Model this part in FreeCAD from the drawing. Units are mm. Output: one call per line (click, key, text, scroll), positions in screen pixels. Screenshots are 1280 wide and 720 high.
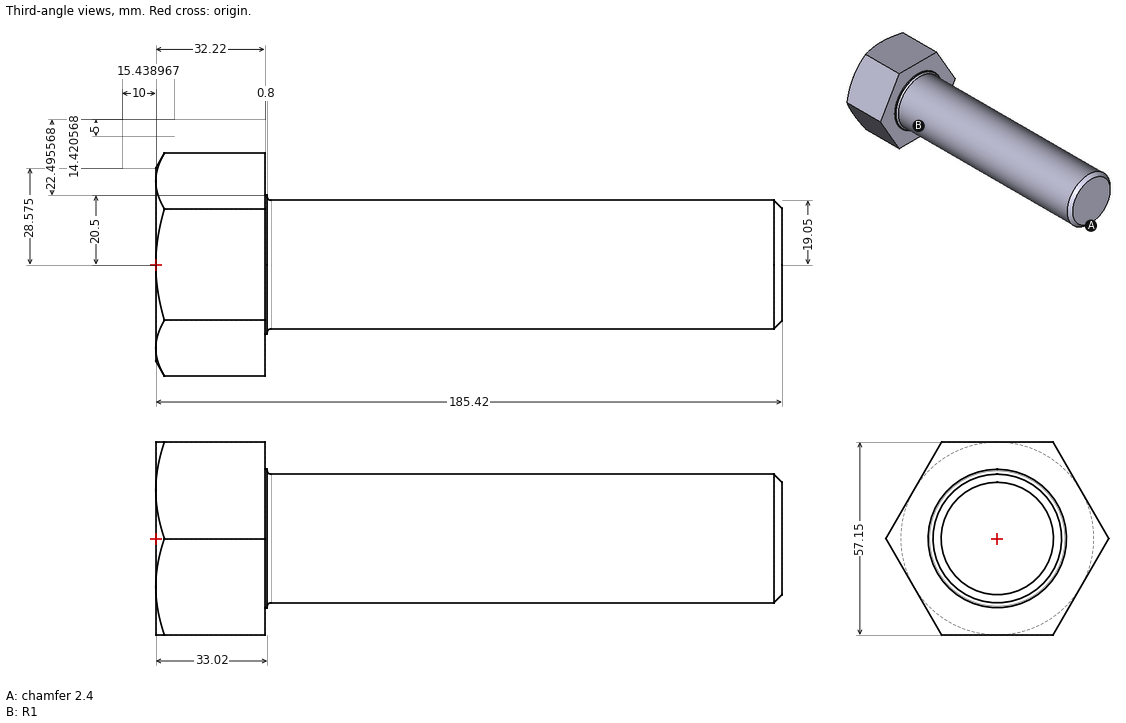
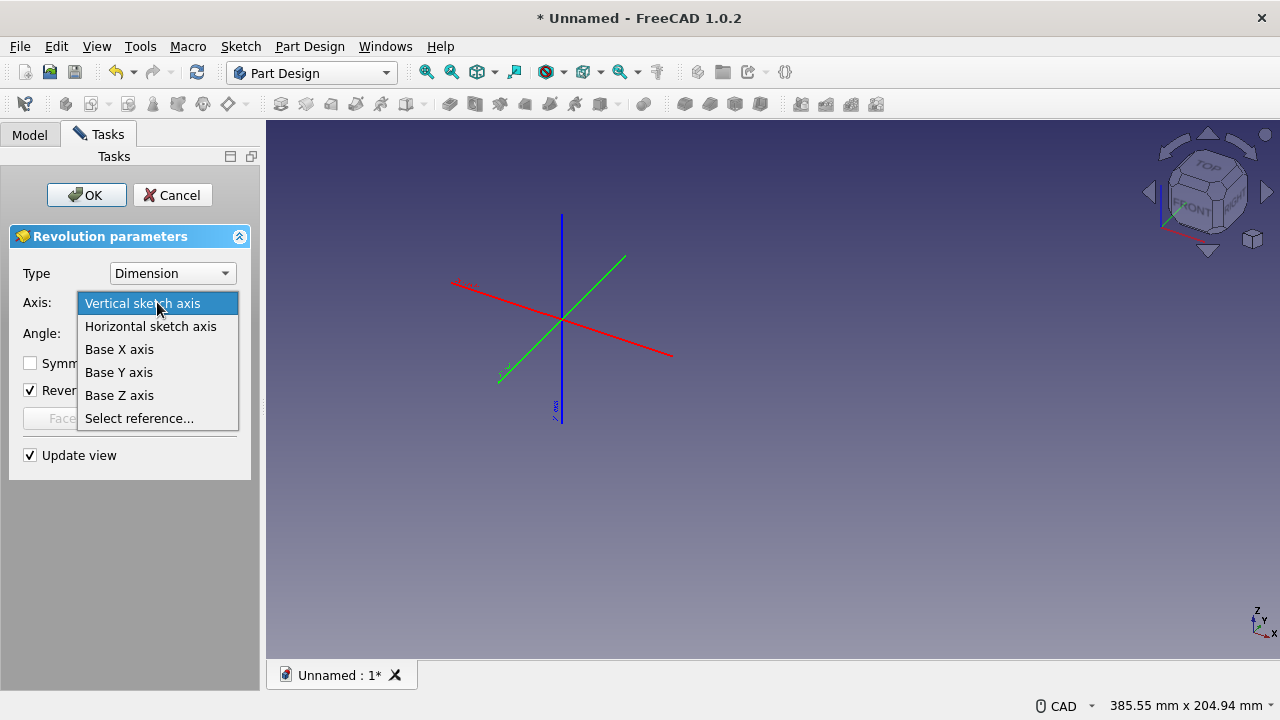
click(156, 326)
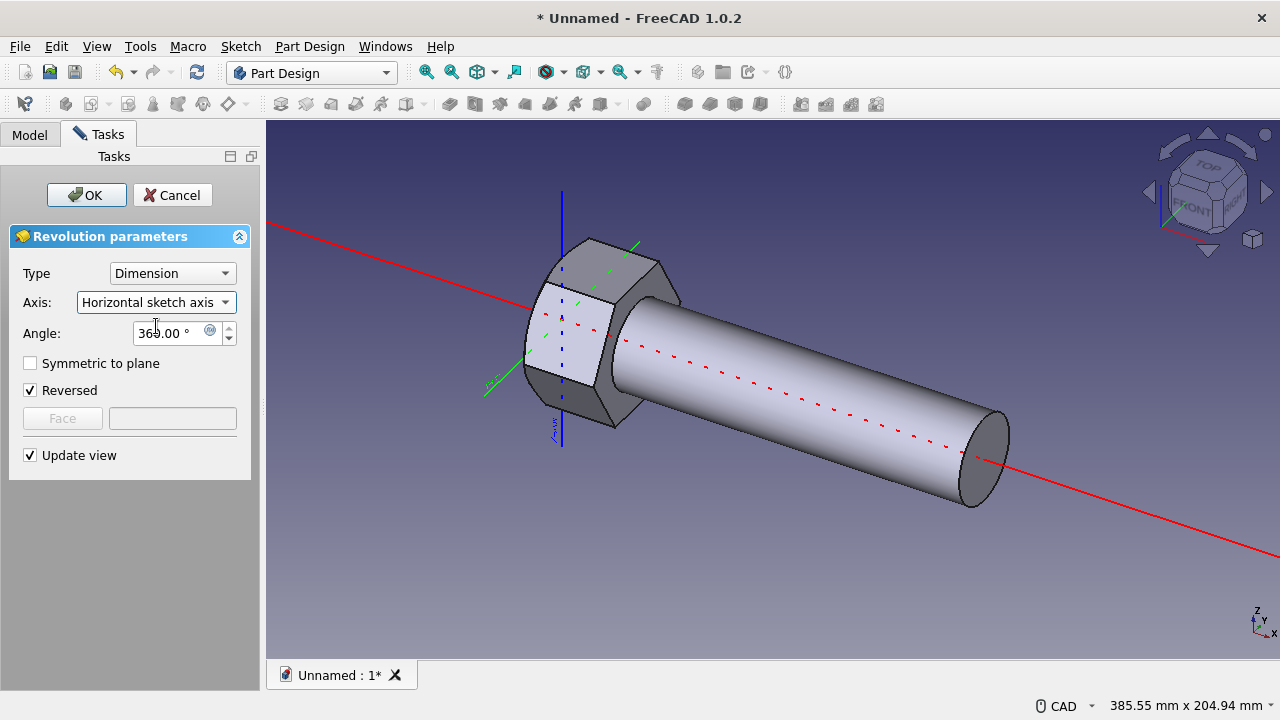
click(87, 195)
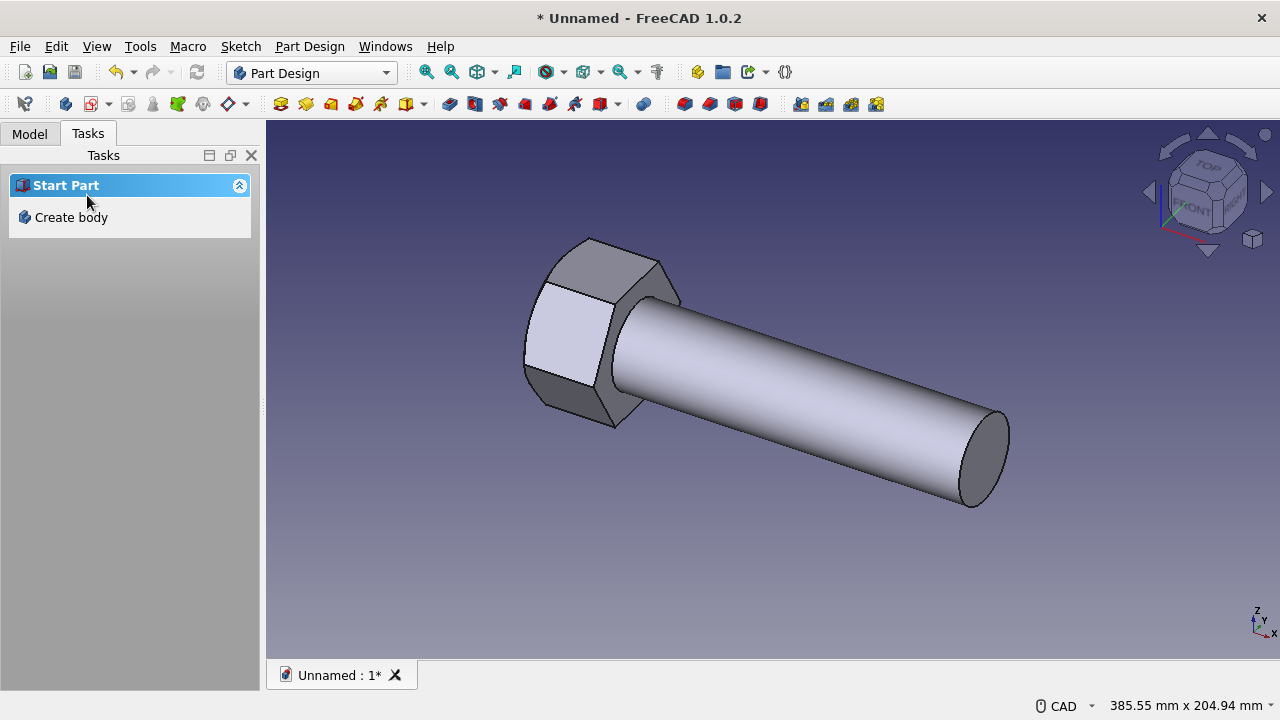
click(90, 104)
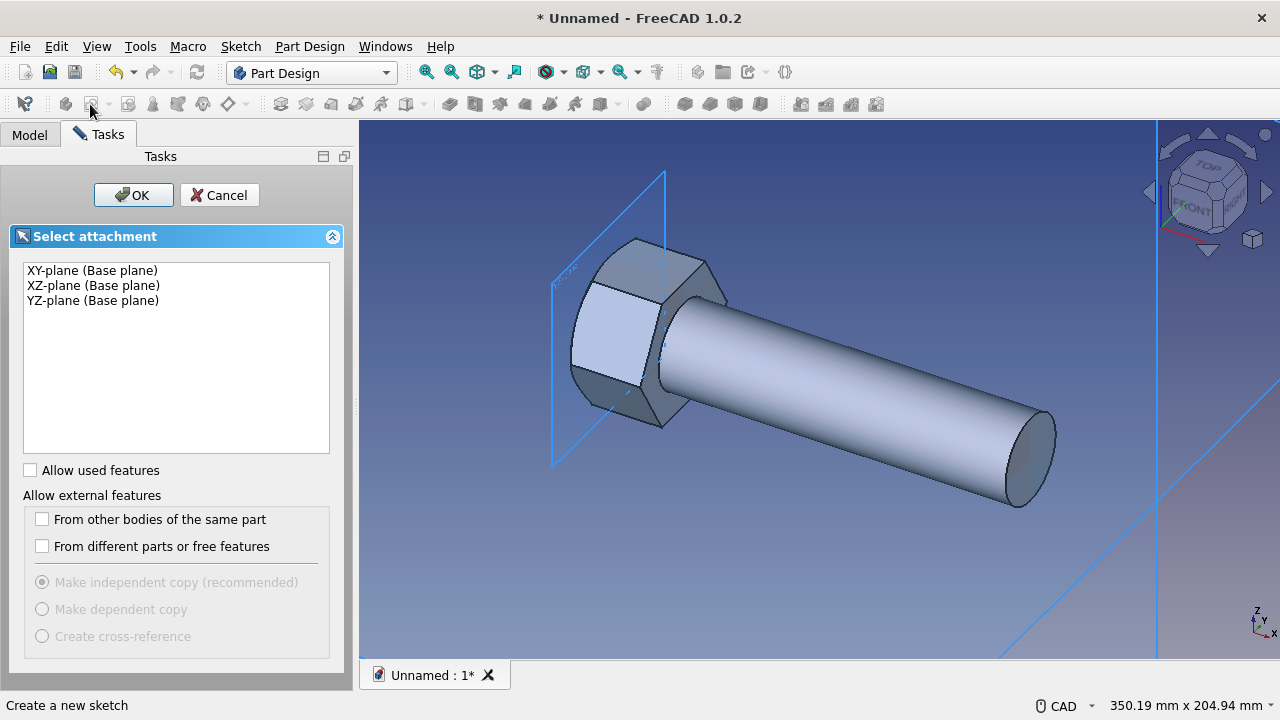
click(84, 270)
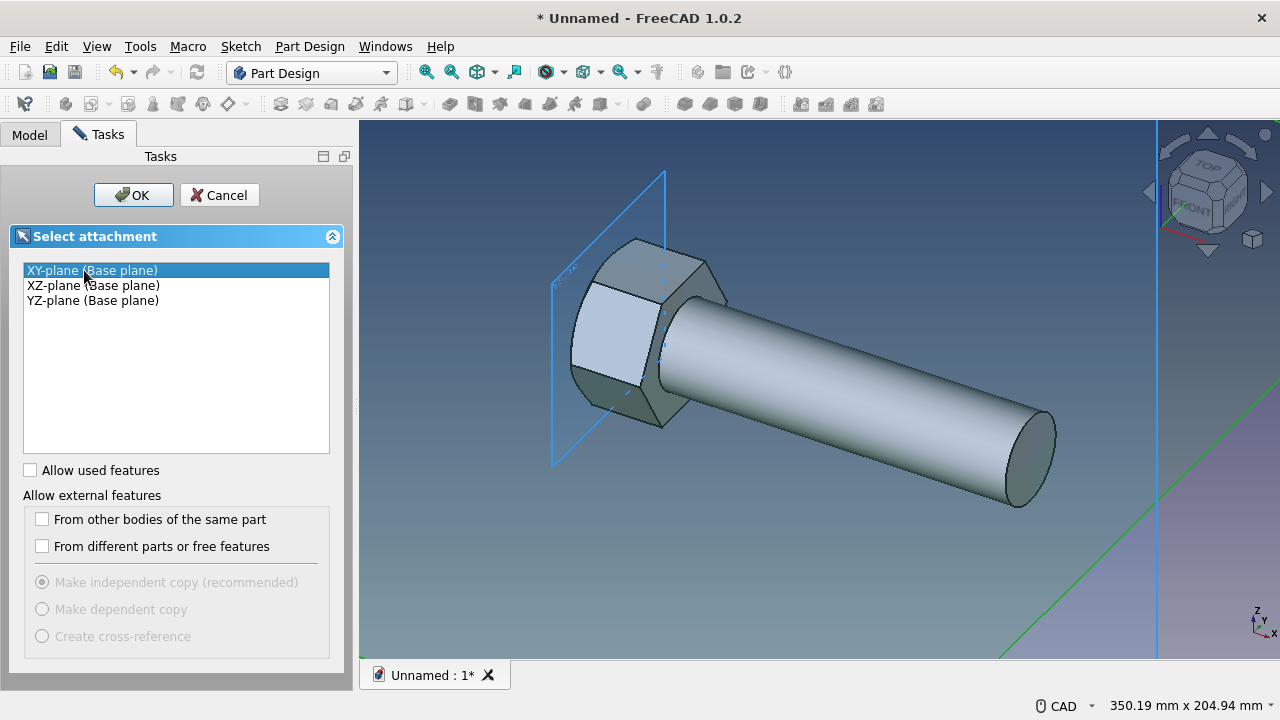
click(134, 195)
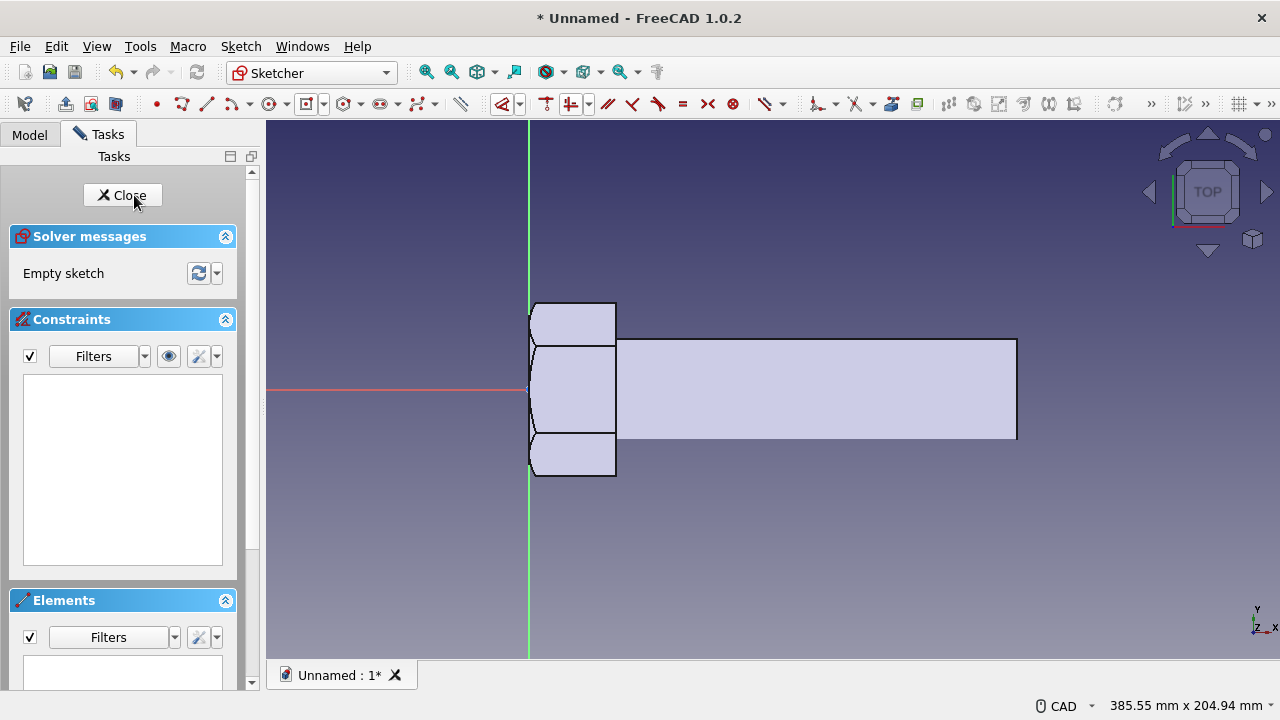
key(q)
key(s)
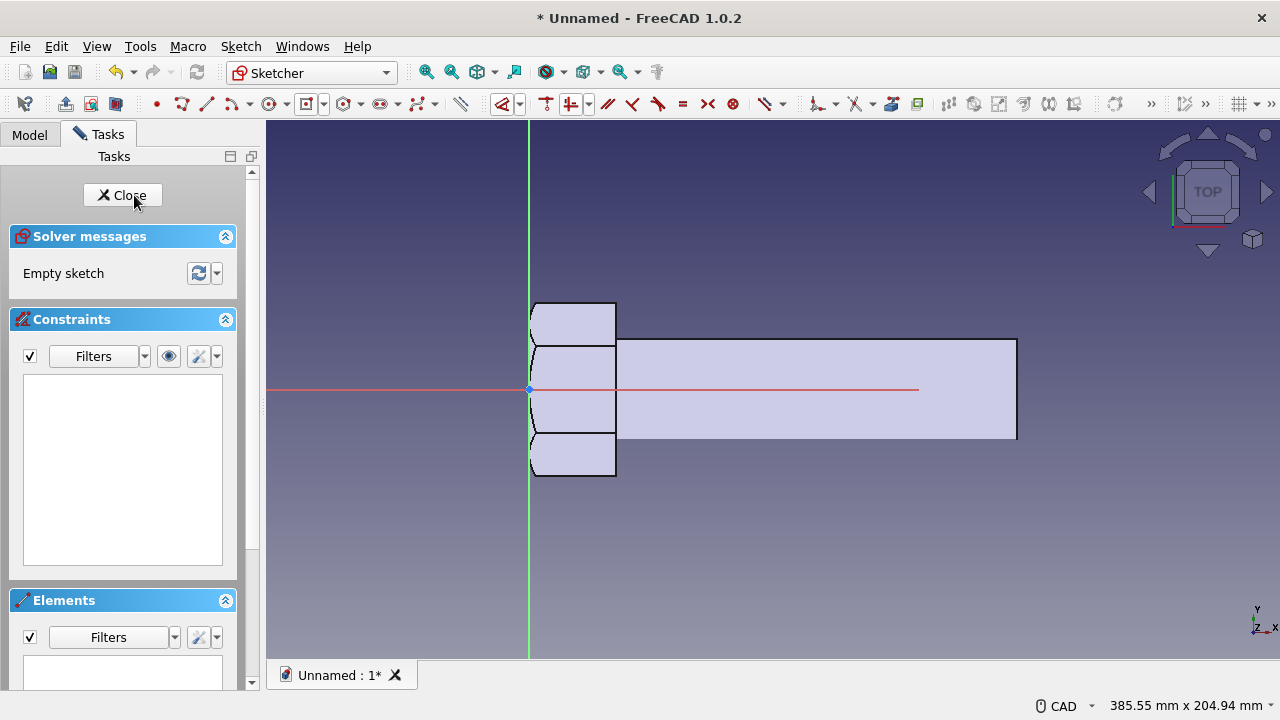
scroll(516, 309, up, 6)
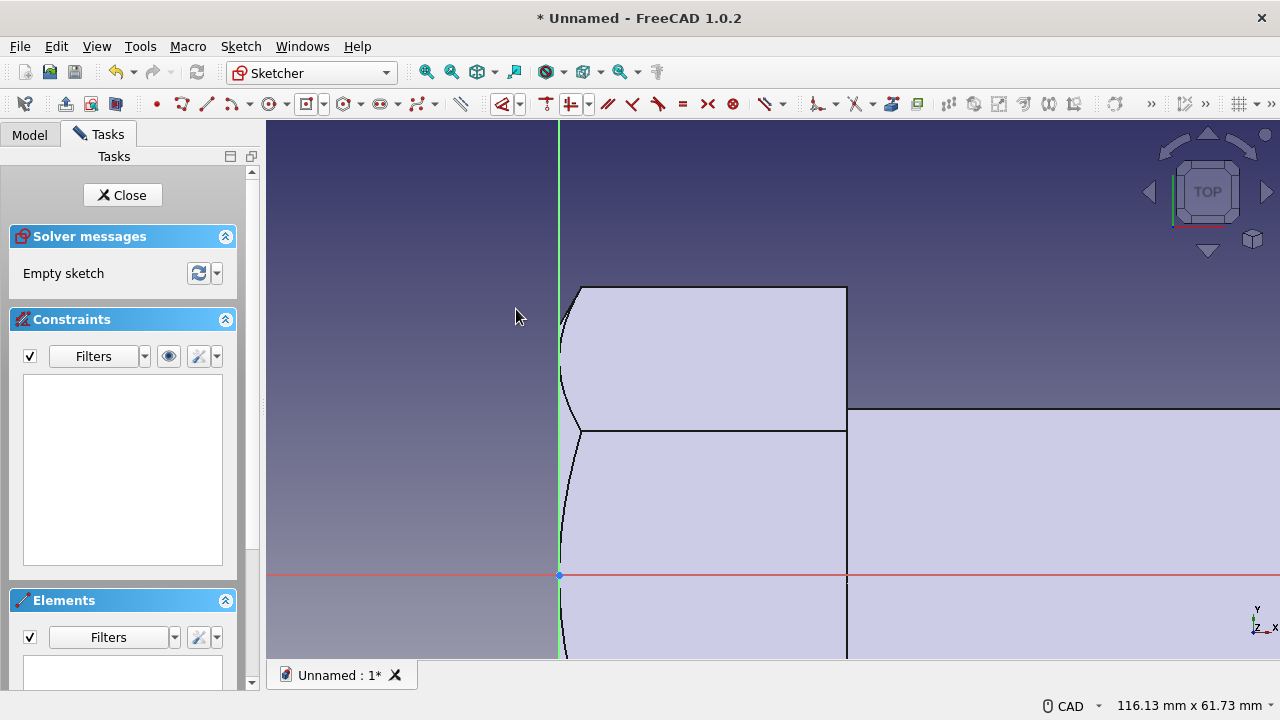
click(324, 104)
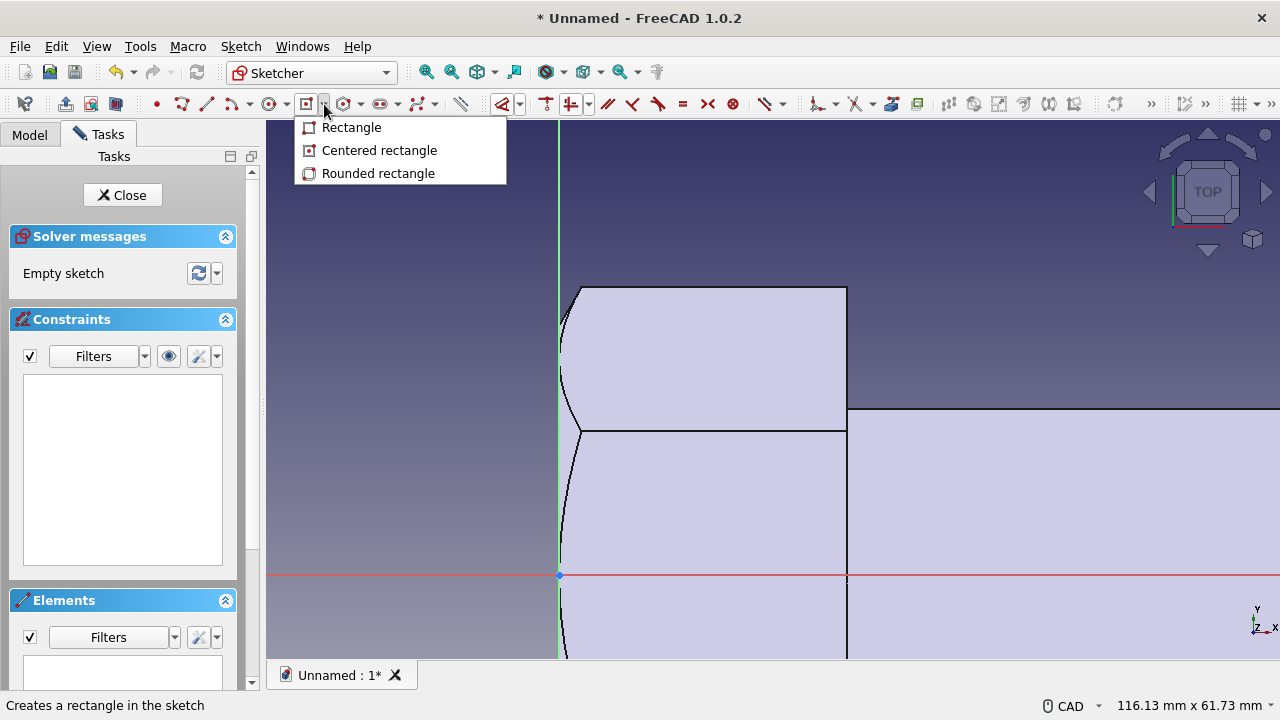
click(400, 128)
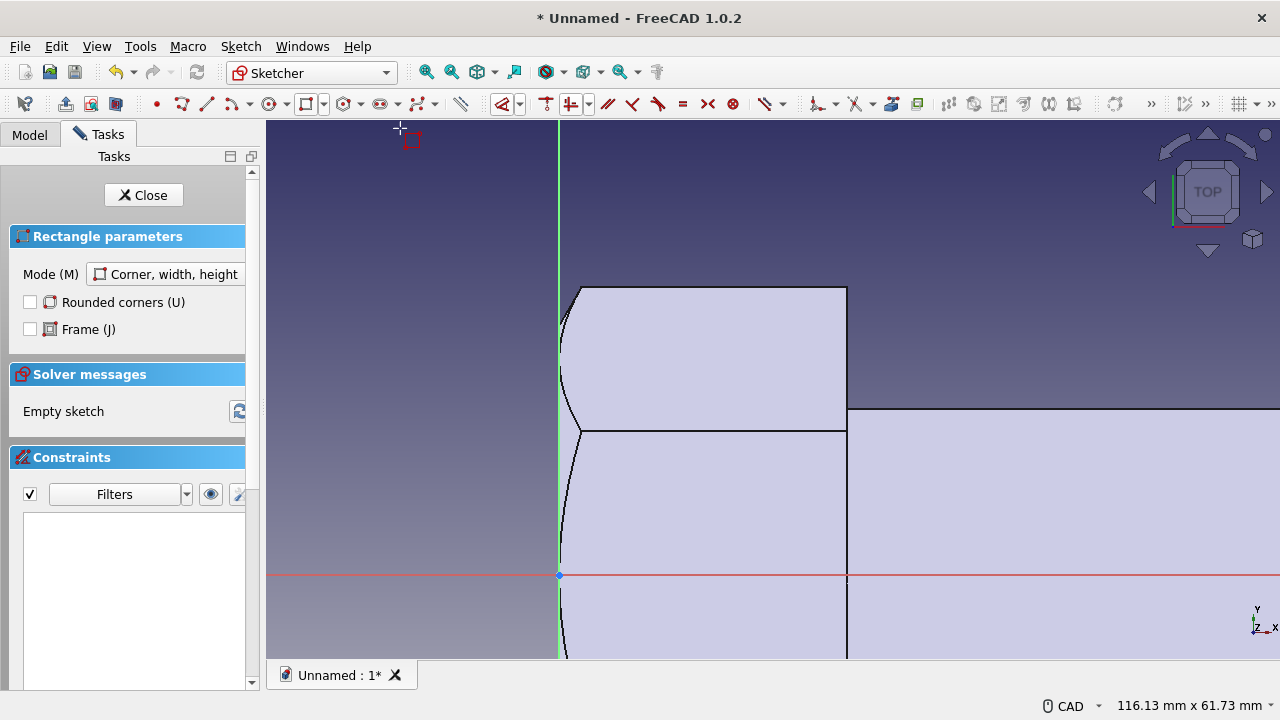
scroll(841, 200, up, 5)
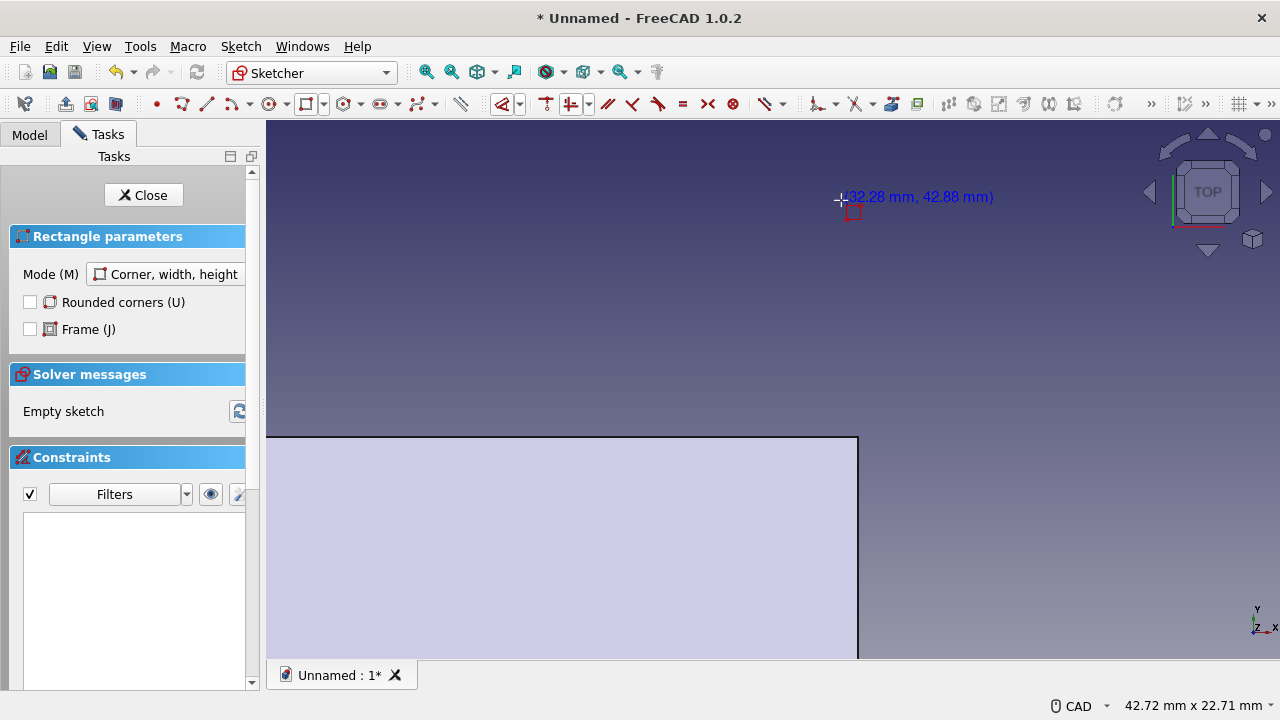
click(839, 200)